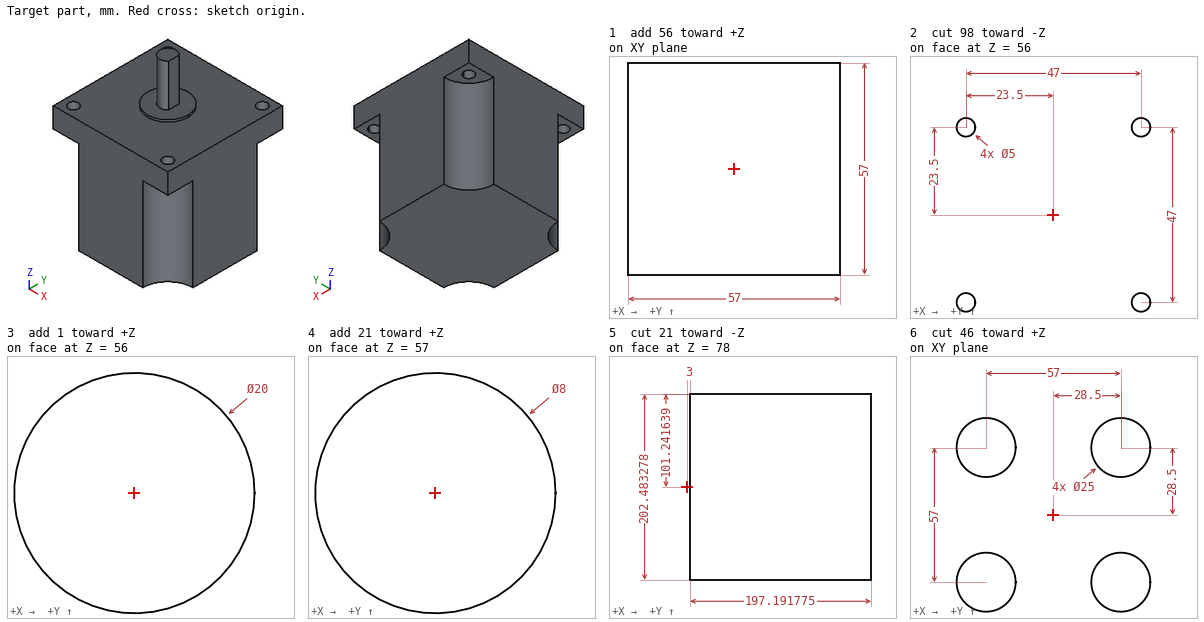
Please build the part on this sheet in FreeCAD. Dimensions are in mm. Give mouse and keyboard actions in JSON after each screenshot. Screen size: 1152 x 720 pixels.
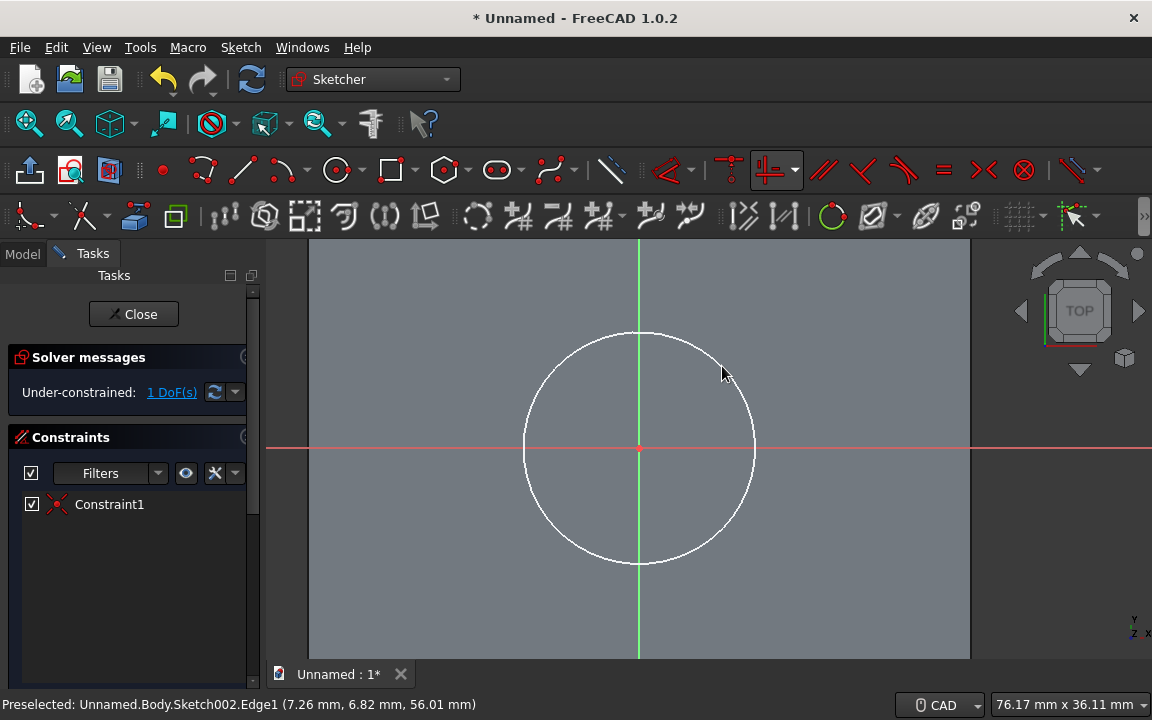
{"action": "left_click", "coordinate": [666, 170]}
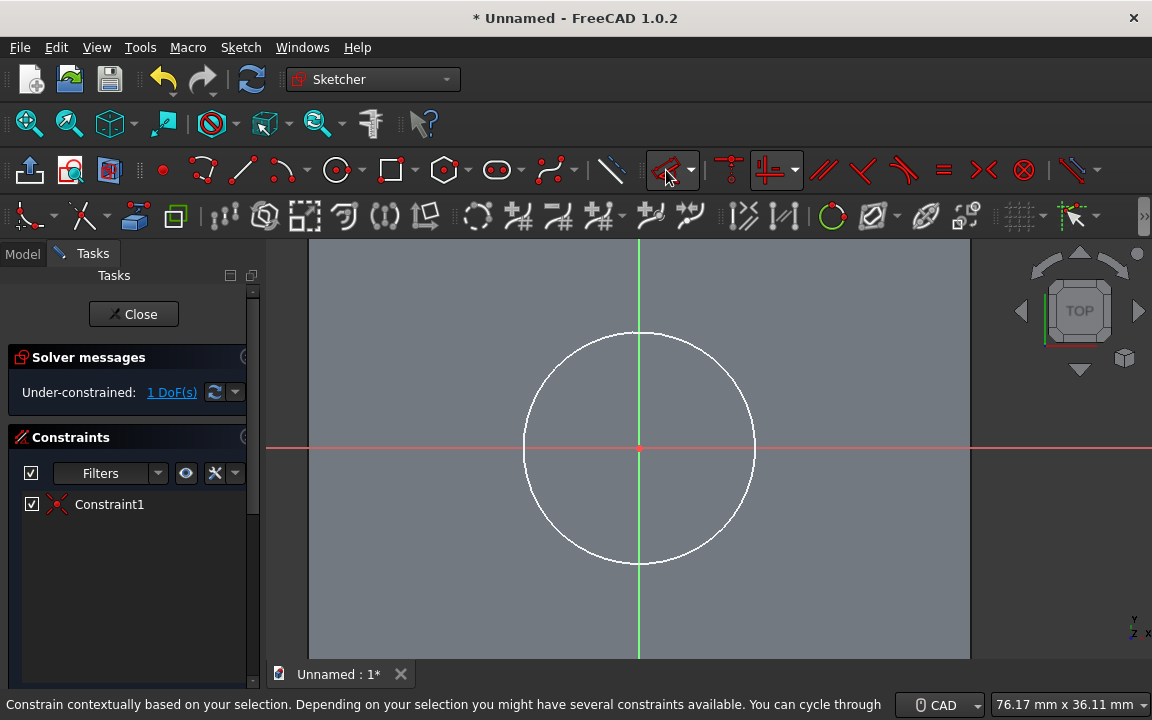
{"action": "left_click", "coordinate": [721, 366]}
{"action": "left_click", "coordinate": [744, 343]}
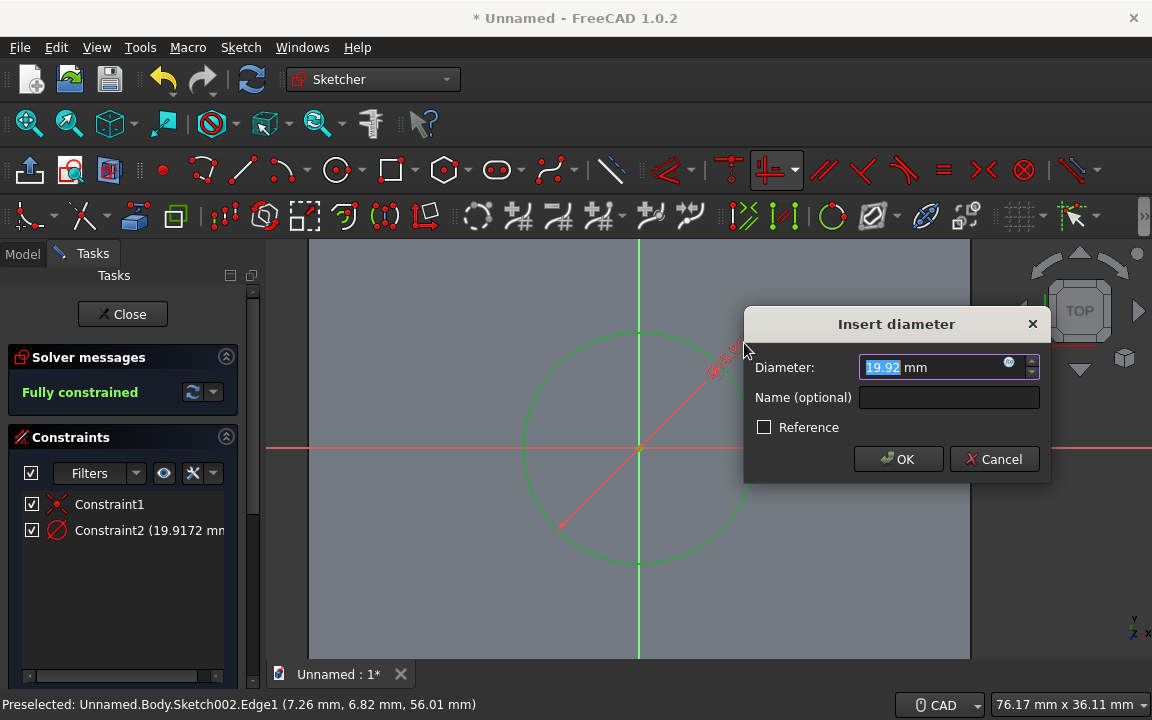
{"action": "type", "text": "20"}
{"action": "key", "text": "Return"}
{"action": "key", "text": "Escape"}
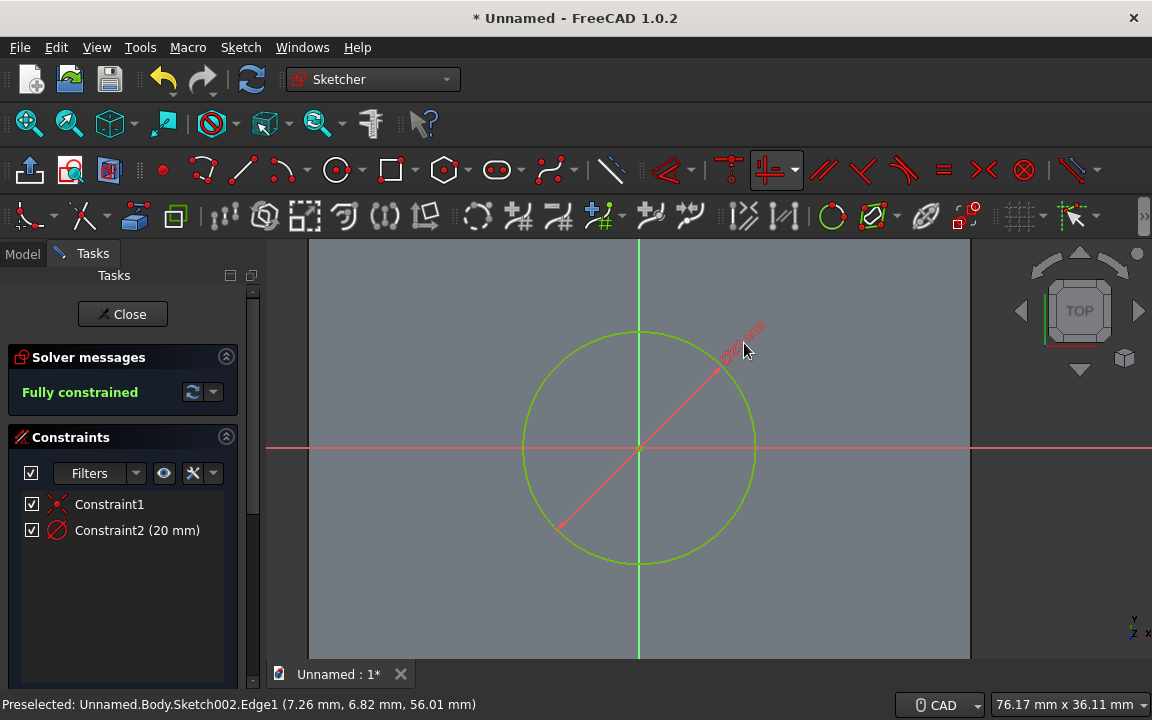
{"action": "left_click", "coordinate": [123, 314]}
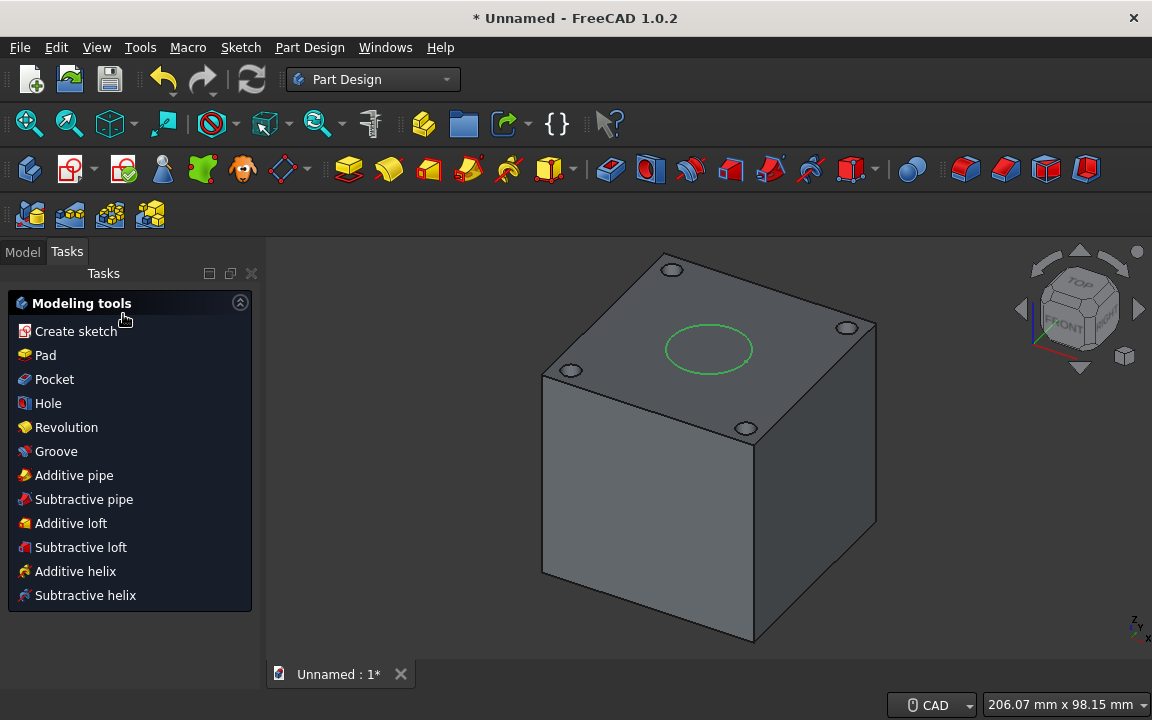
{"action": "left_click", "coordinate": [350, 170]}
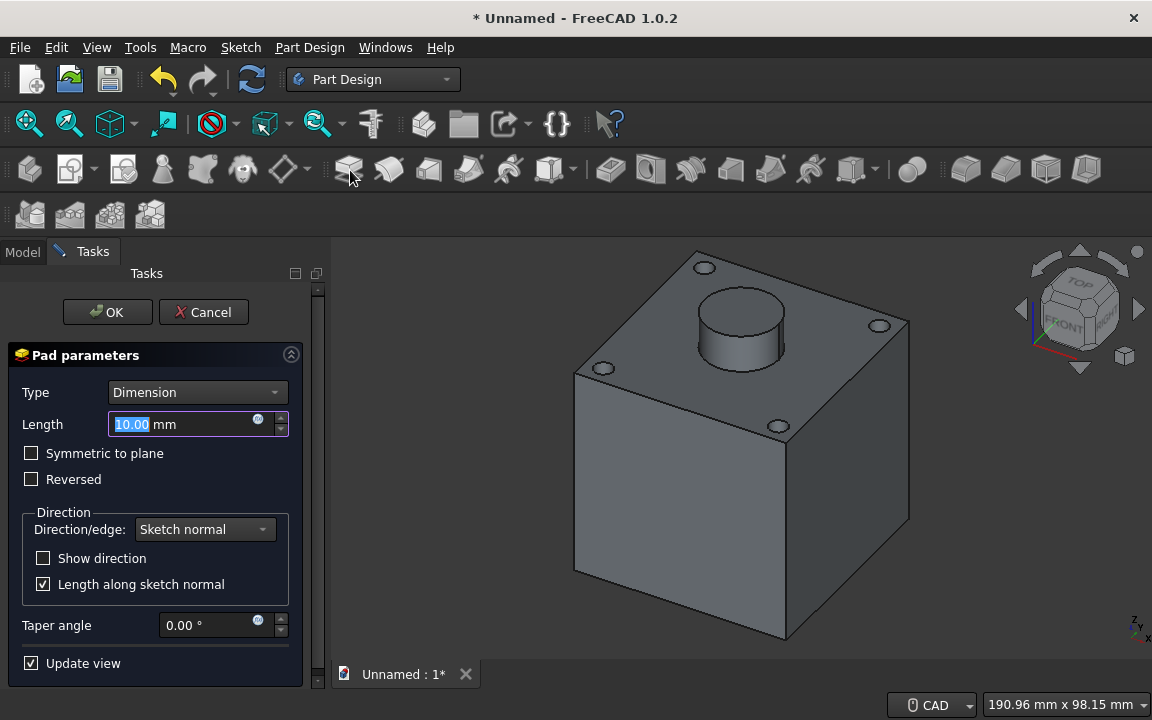
{"action": "type", "text": "1"}
{"action": "key", "text": "Tab"}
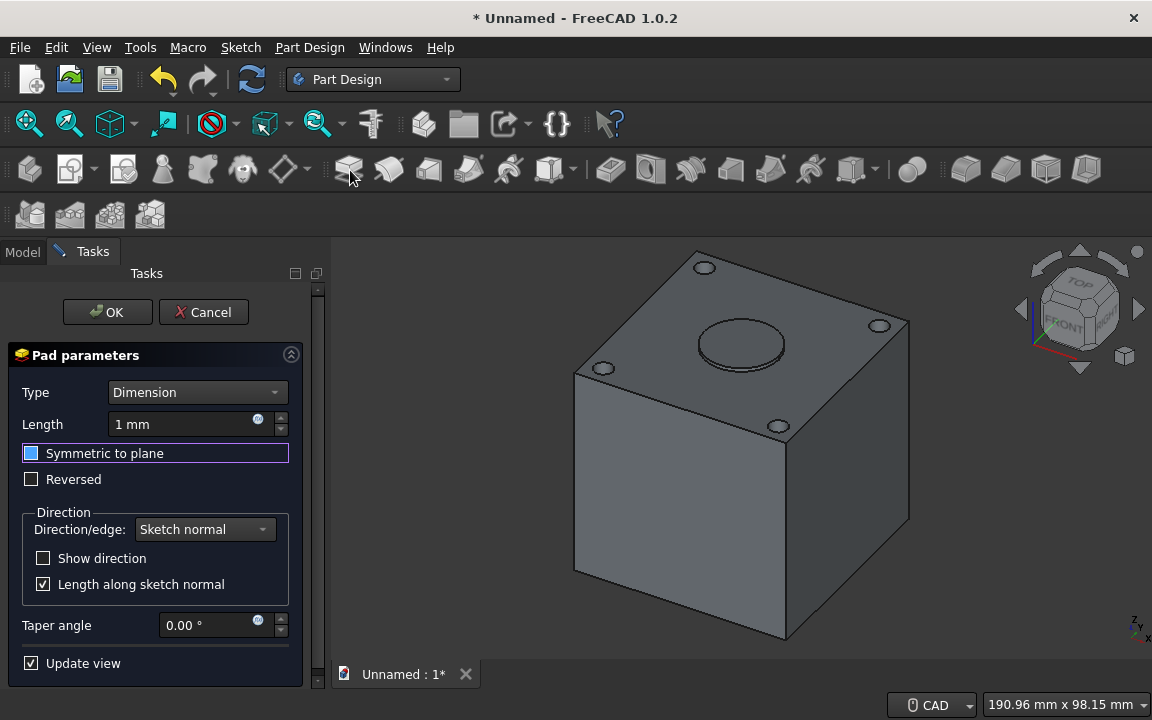
{"action": "left_click", "coordinate": [108, 312]}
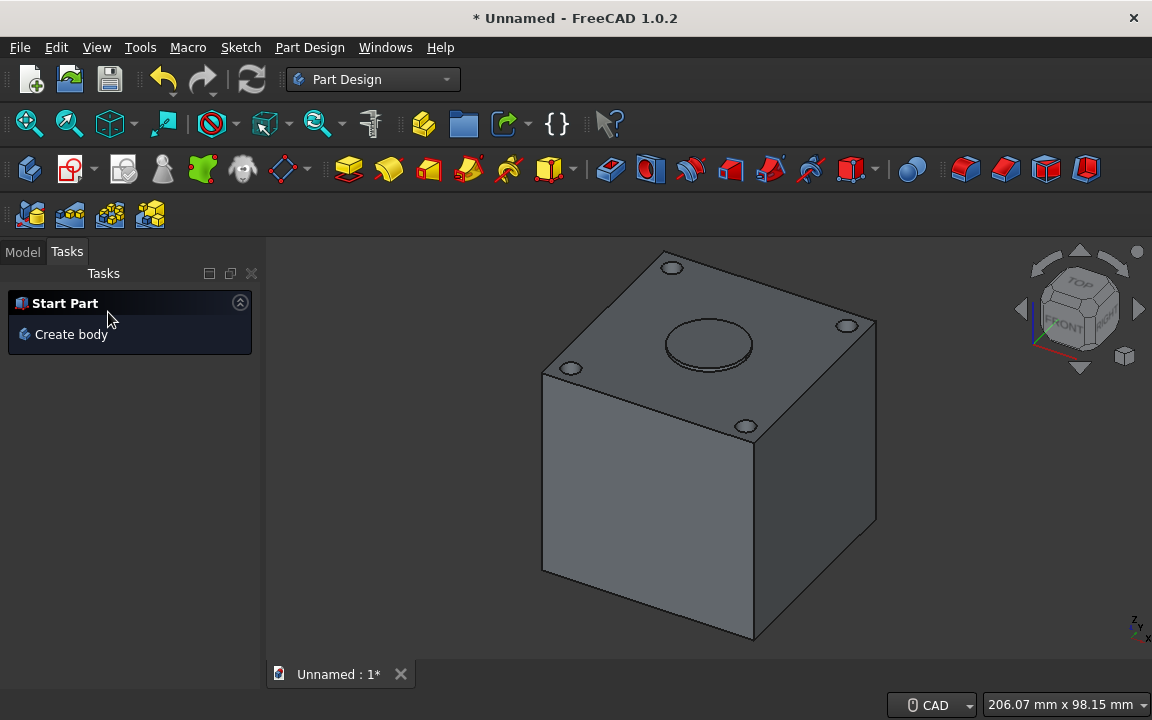
{"action": "left_click", "coordinate": [709, 343]}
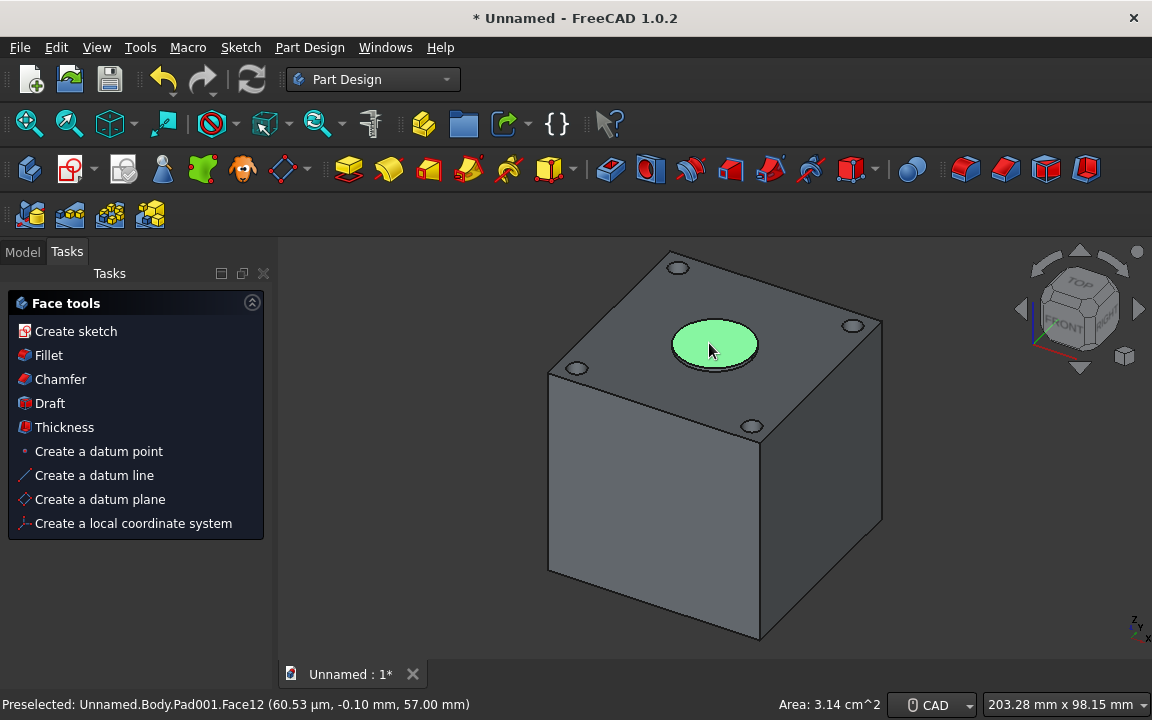
{"action": "left_click", "coordinate": [70, 170]}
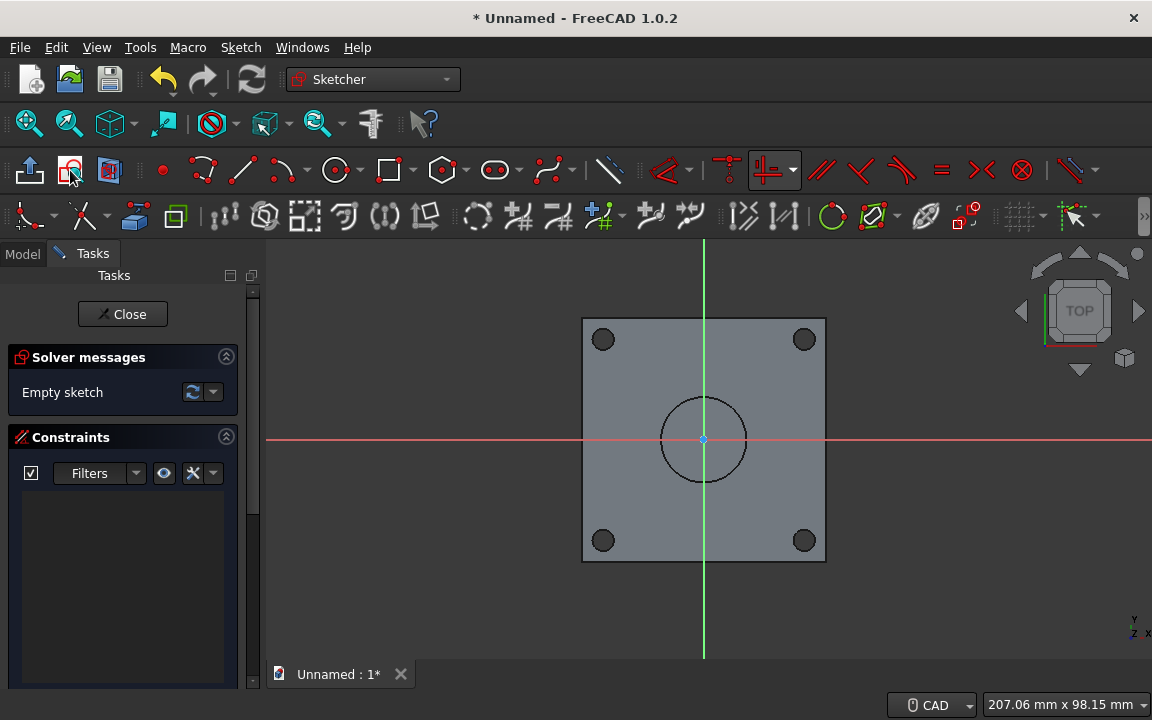
{"action": "scroll", "coordinate": [714, 438], "scroll_direction": "up", "scroll_amount": 10}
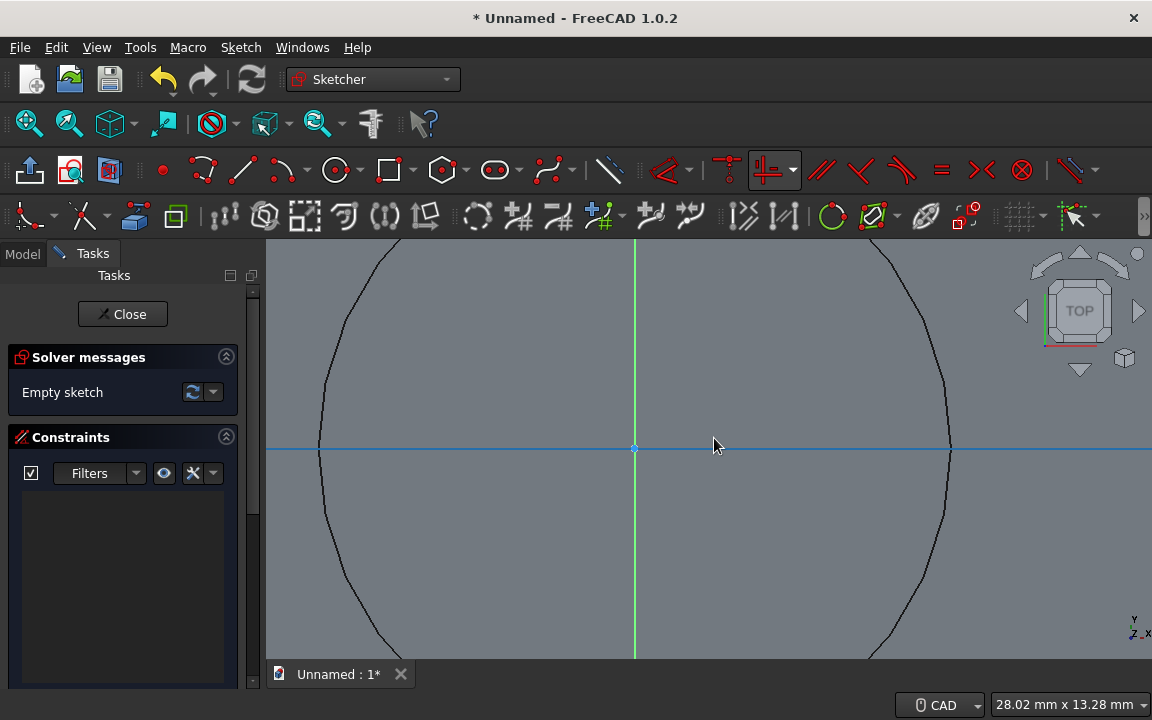
{"action": "left_click", "coordinate": [336, 170]}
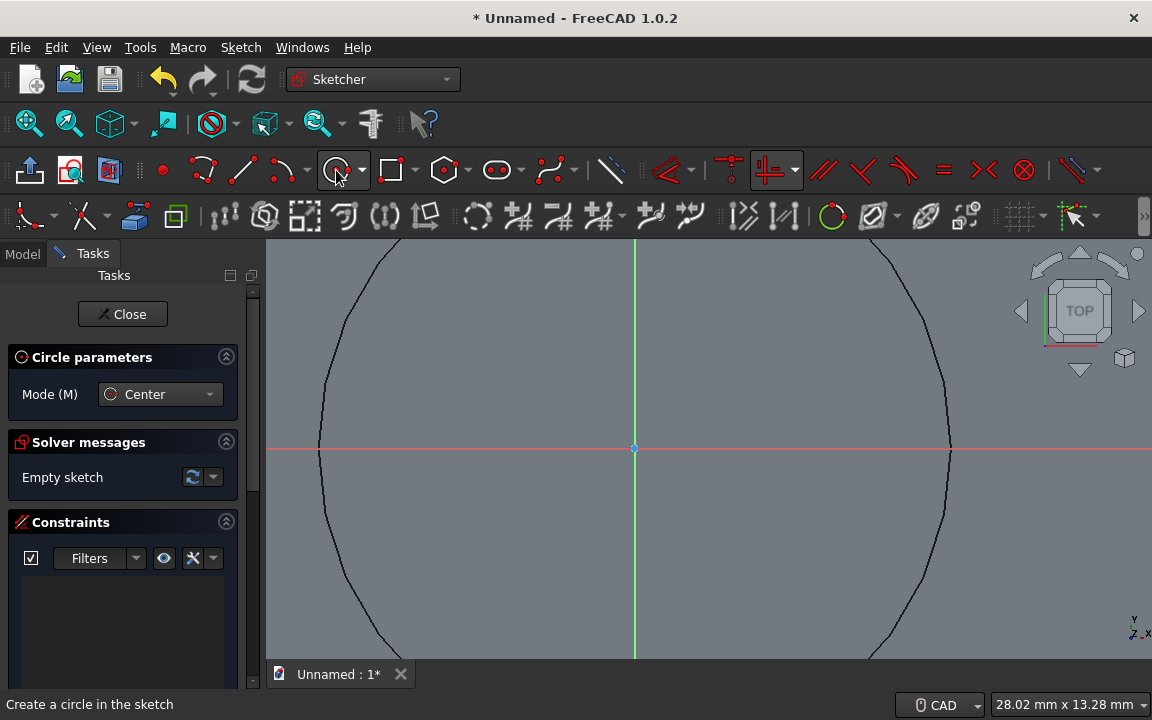
{"action": "left_click", "coordinate": [635, 449]}
{"action": "left_click", "coordinate": [724, 359]}
{"action": "key", "text": "Escape"}